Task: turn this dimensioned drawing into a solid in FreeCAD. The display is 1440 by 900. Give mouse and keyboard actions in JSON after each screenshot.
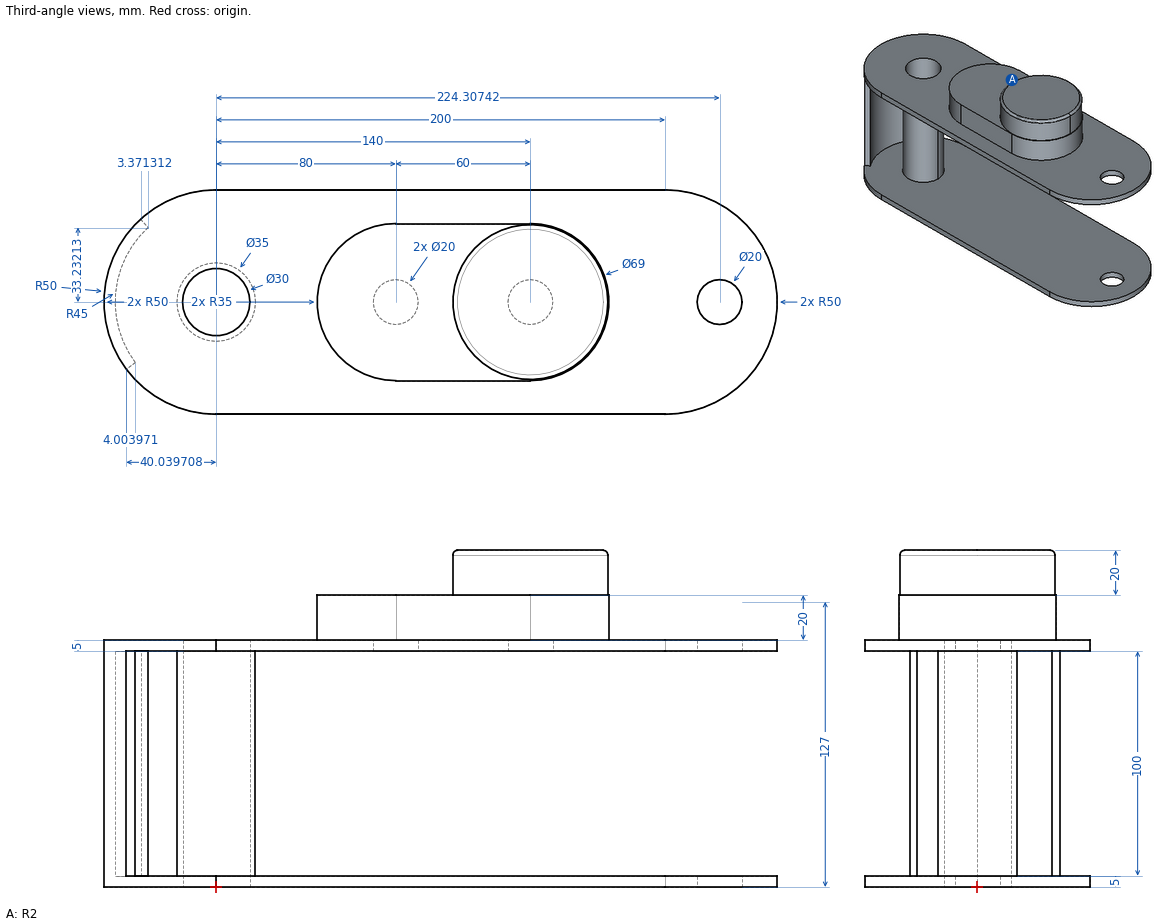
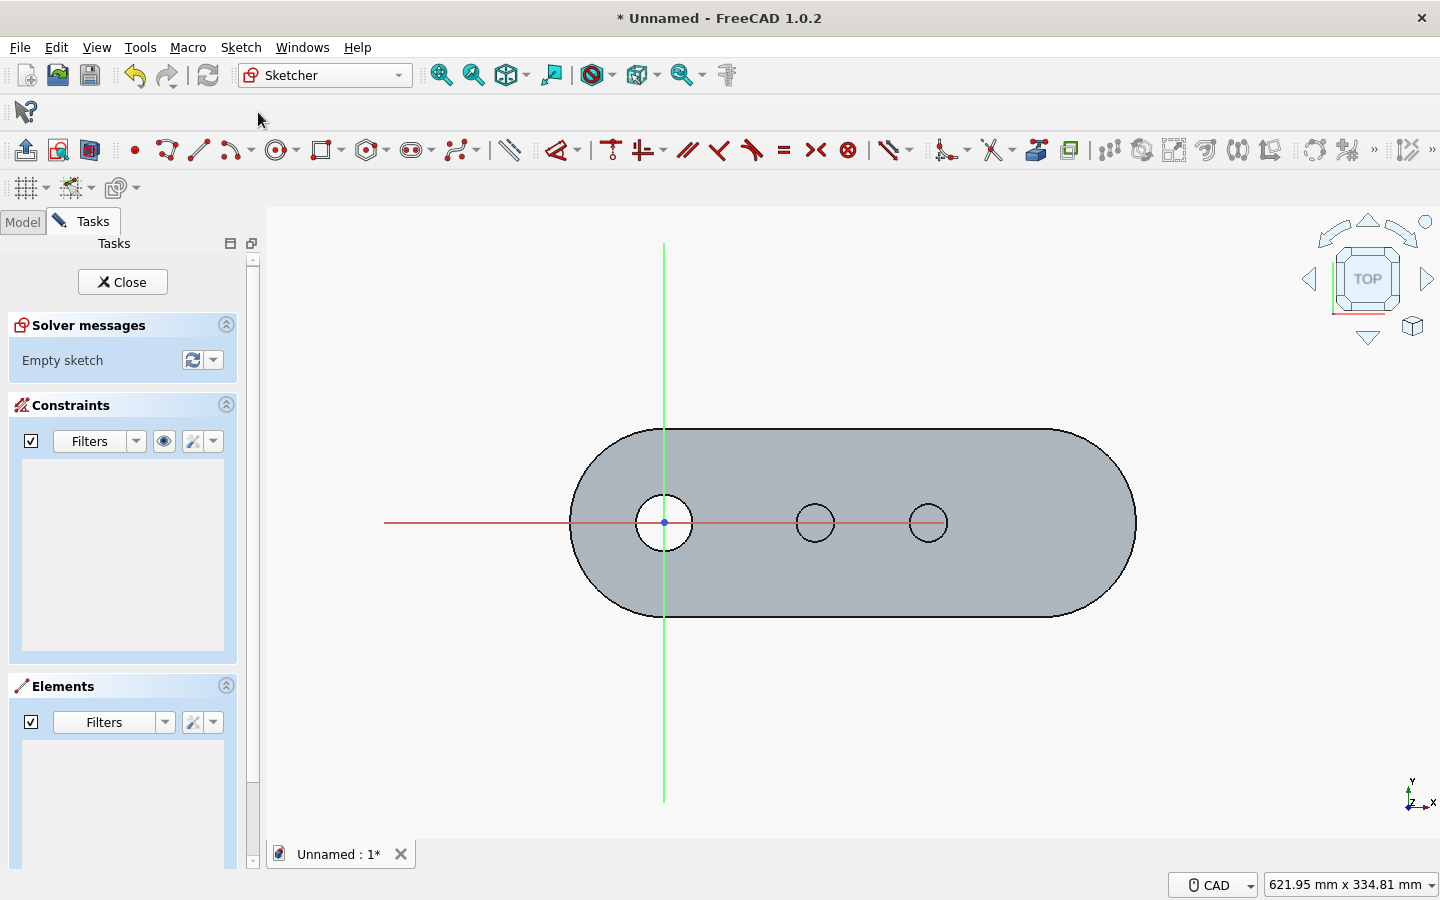
{"action": "scroll", "coordinate": [866, 523], "scroll_direction": "up", "scroll_amount": 4}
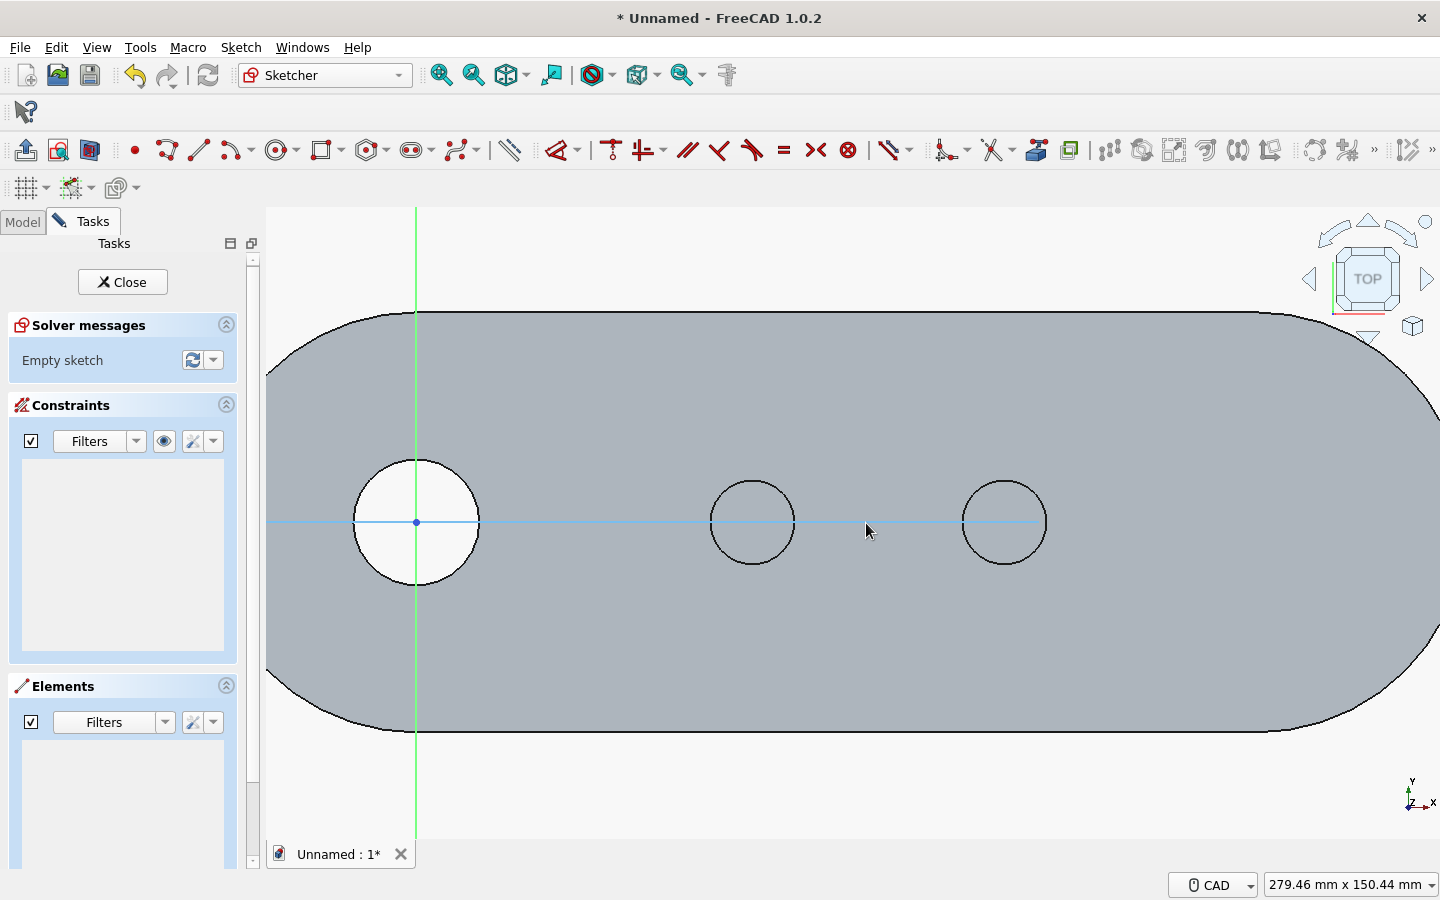
{"action": "left_click", "coordinate": [412, 150]}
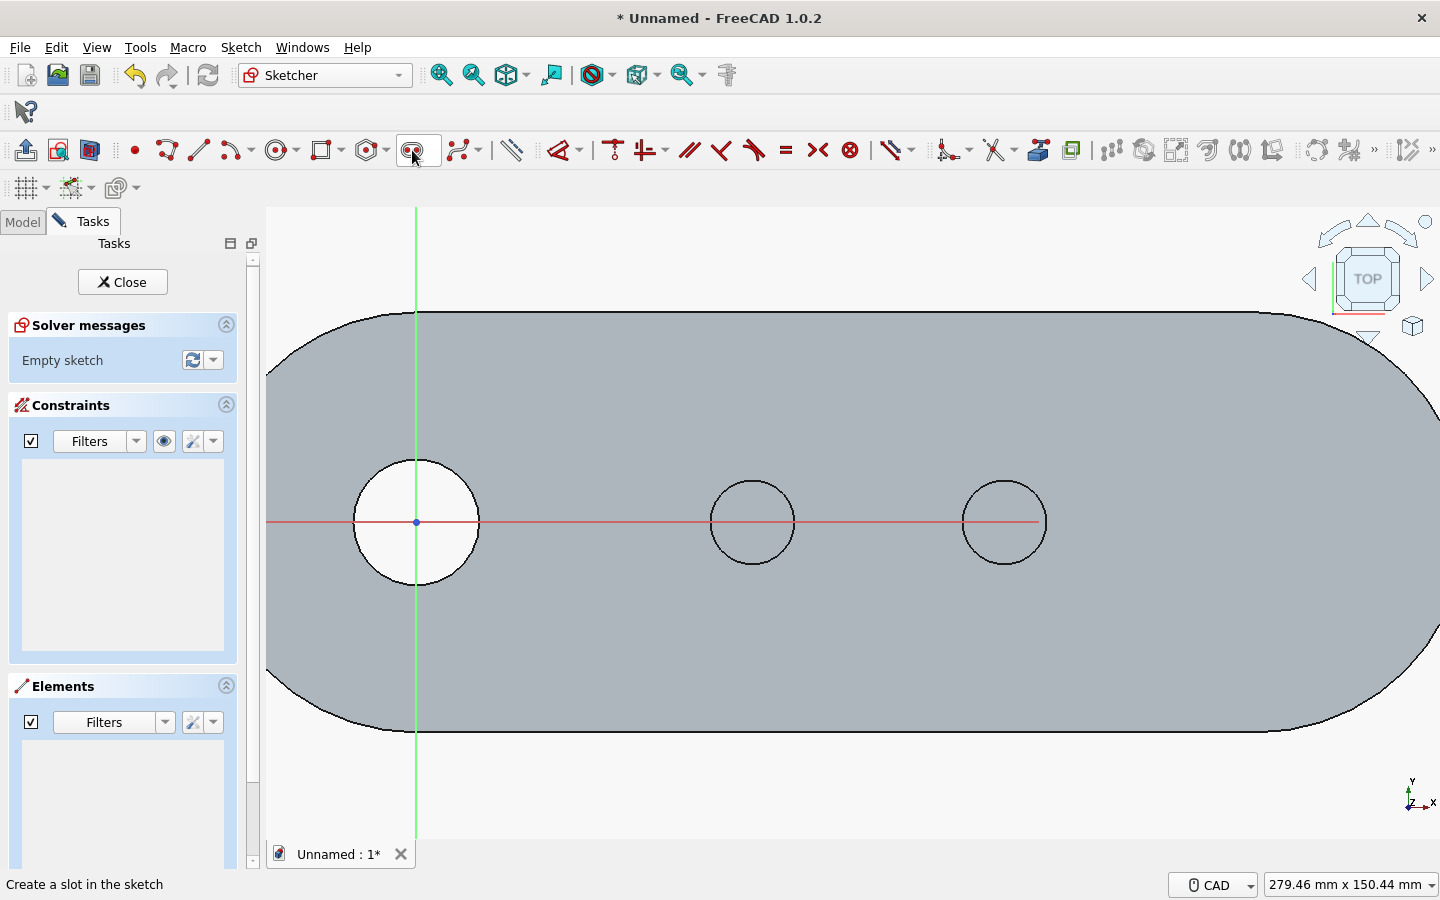
{"action": "left_click", "coordinate": [752, 522]}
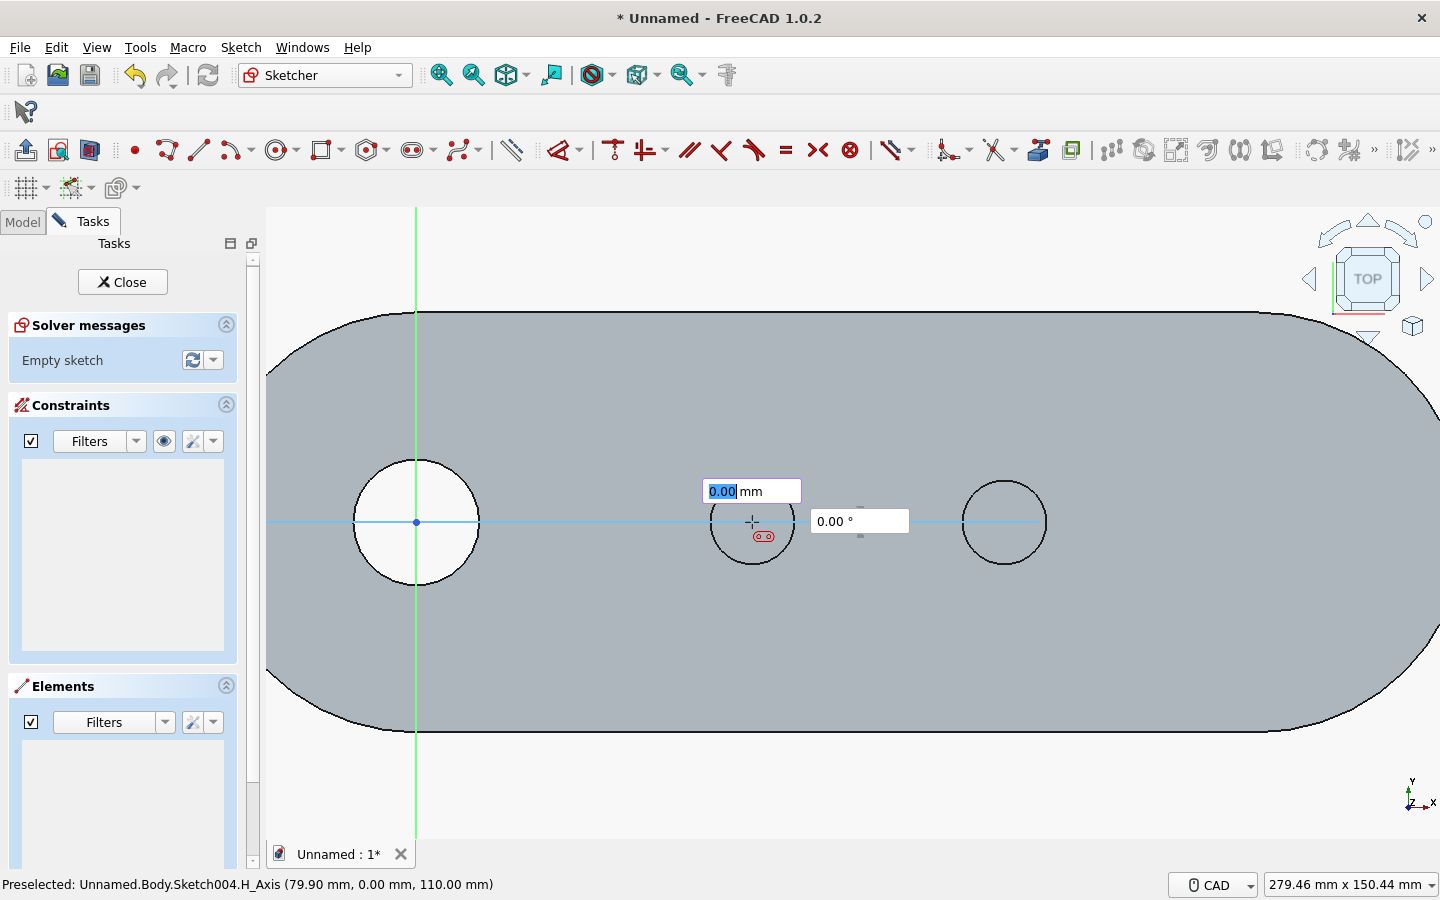
{"action": "left_click", "coordinate": [1004, 513]}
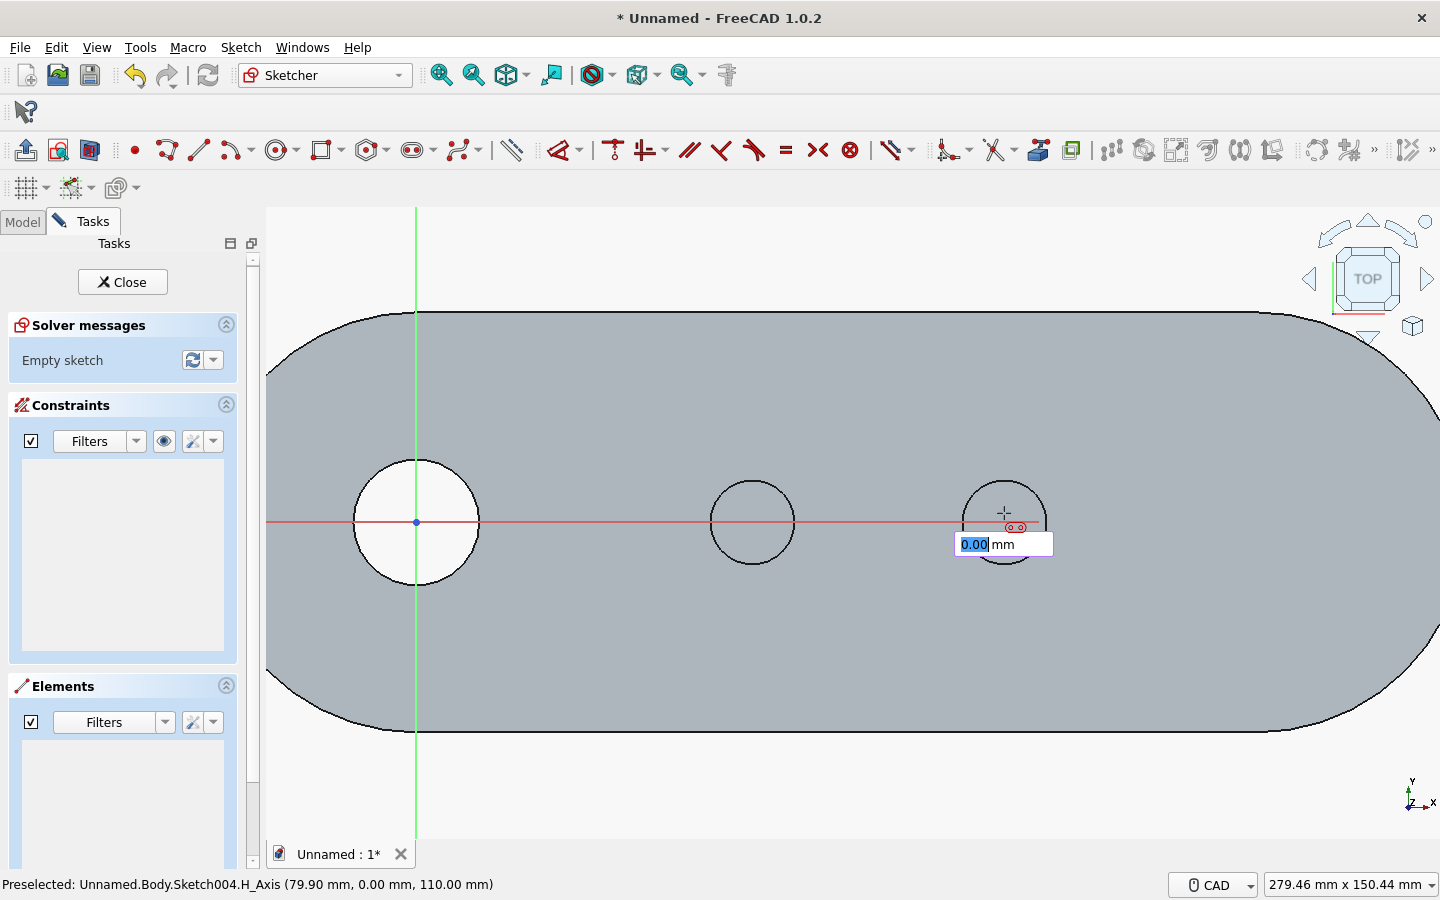
{"action": "left_click", "coordinate": [878, 375]}
{"action": "key", "text": "Escape"}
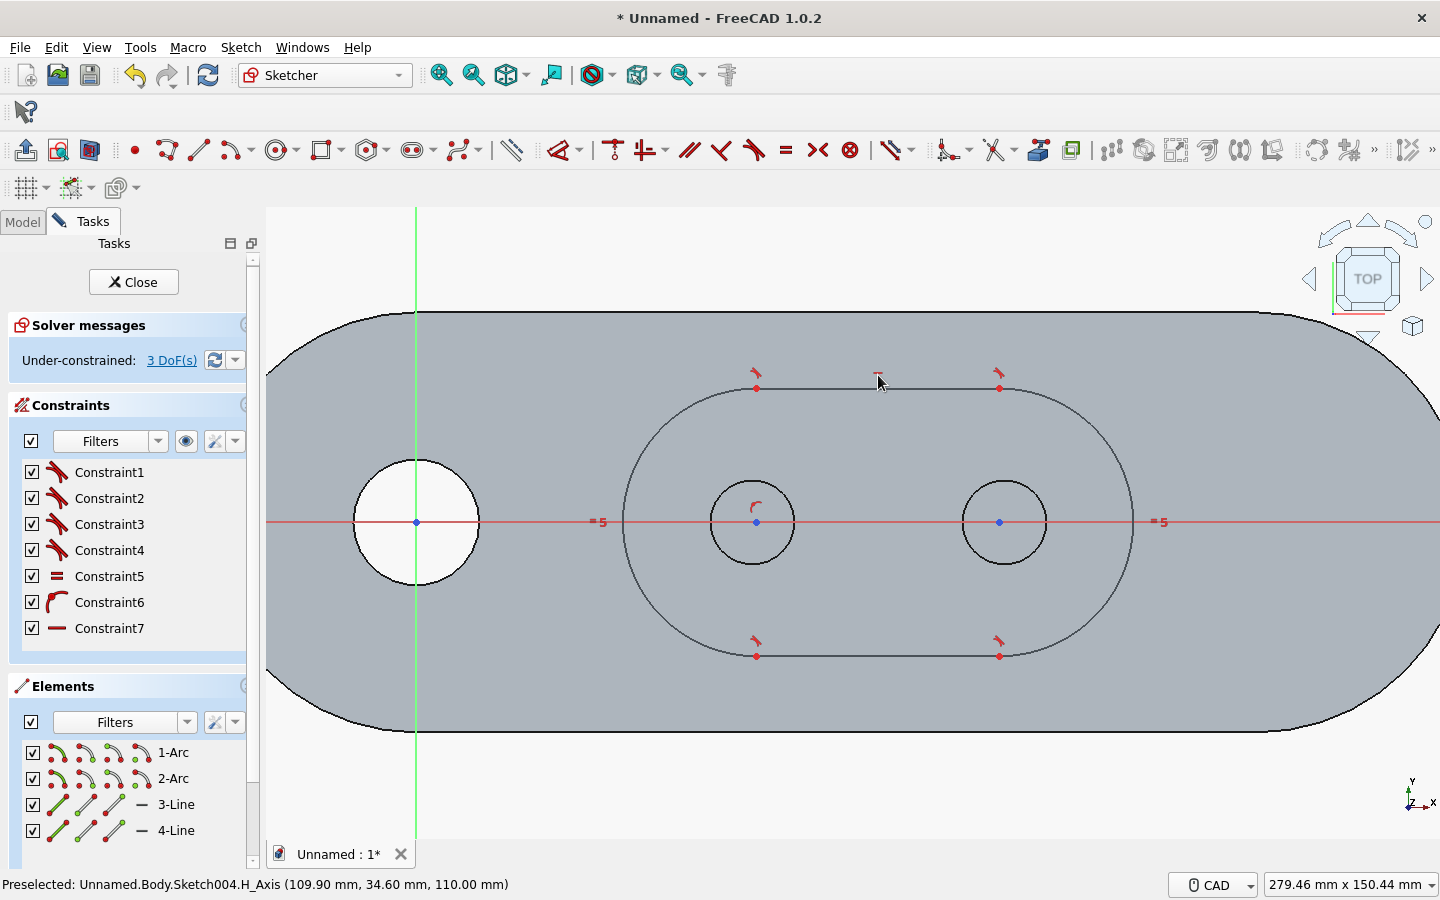
{"action": "left_click", "coordinate": [558, 150]}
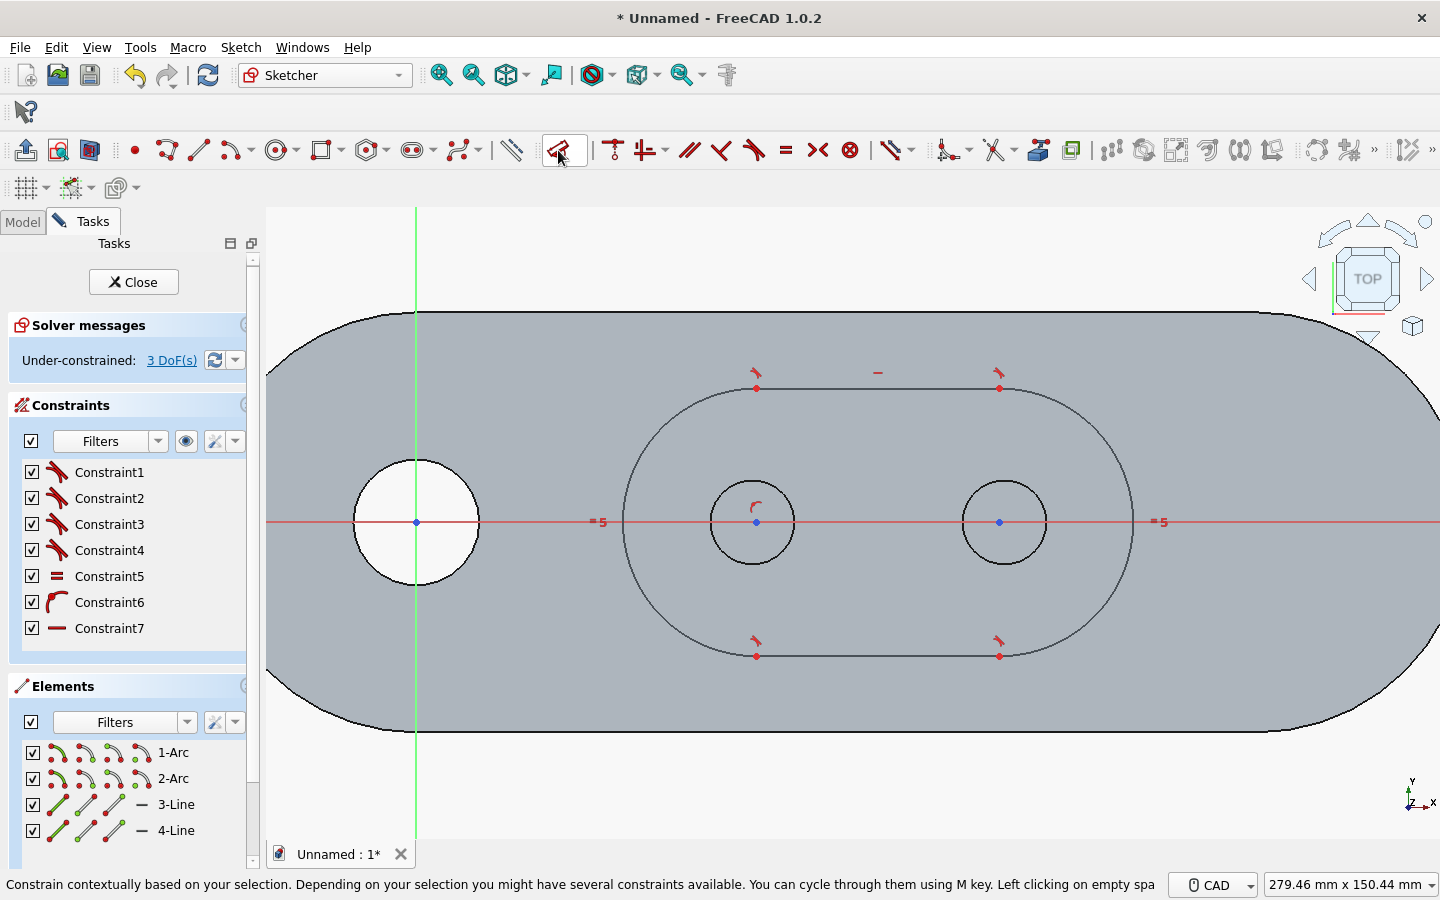
{"action": "left_click", "coordinate": [648, 444]}
{"action": "left_click", "coordinate": [622, 425]}